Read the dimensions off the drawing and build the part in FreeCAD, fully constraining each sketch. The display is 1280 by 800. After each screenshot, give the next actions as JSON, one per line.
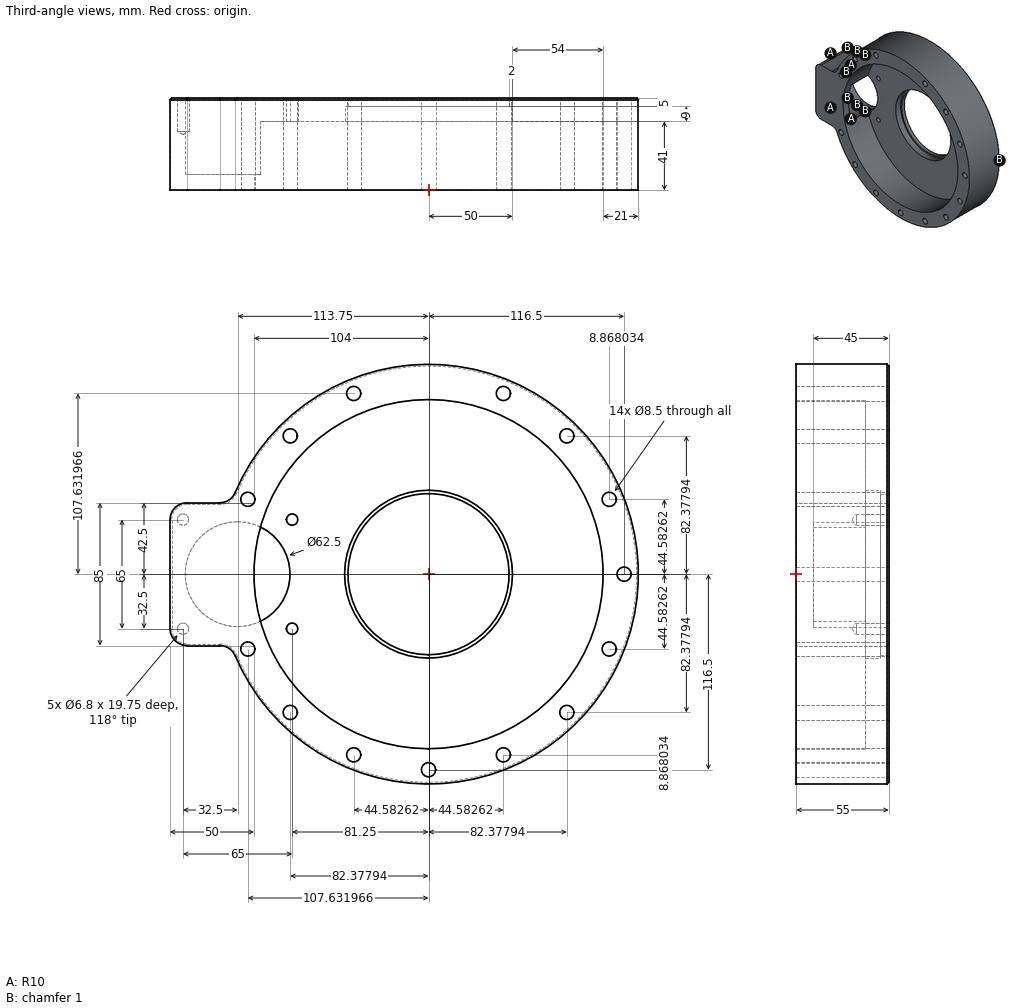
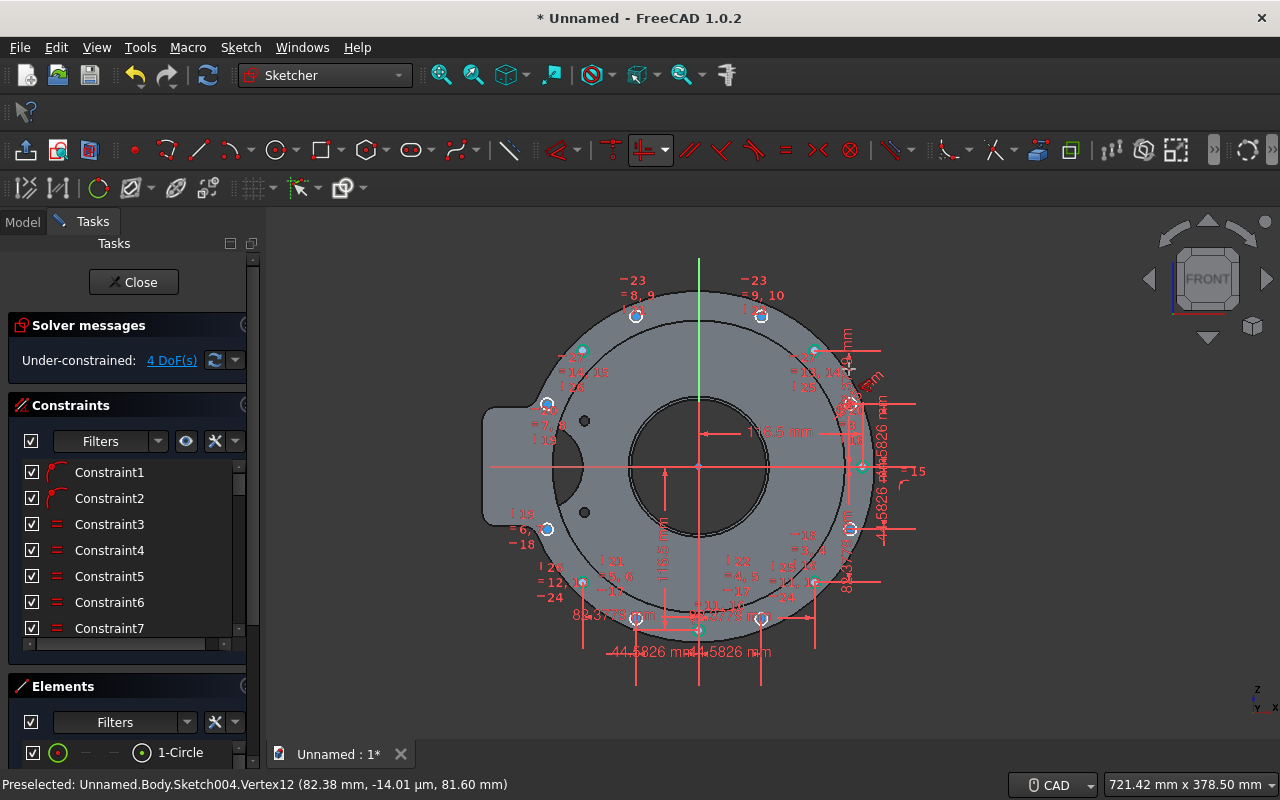
{"action": "scroll", "coordinate": [761, 619], "scroll_direction": "up", "scroll_amount": 6}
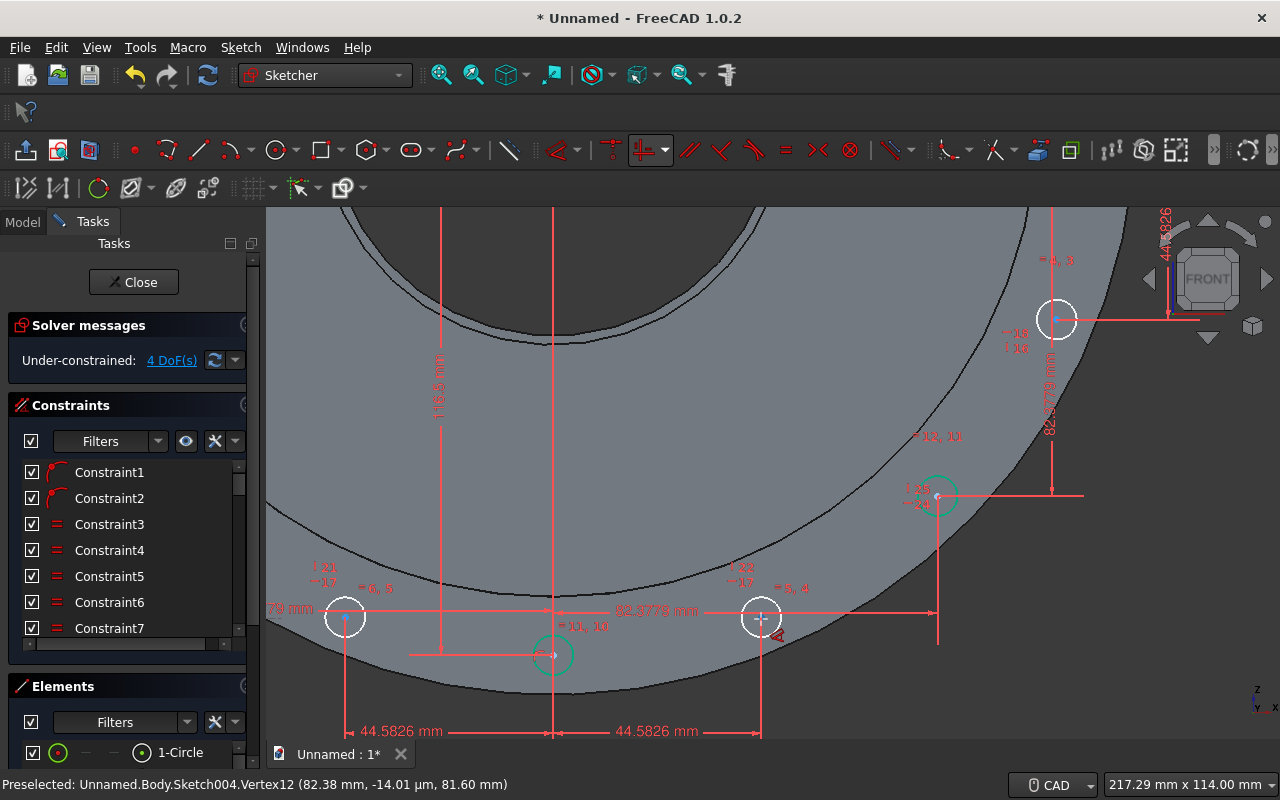
{"action": "left_click", "coordinate": [761, 617]}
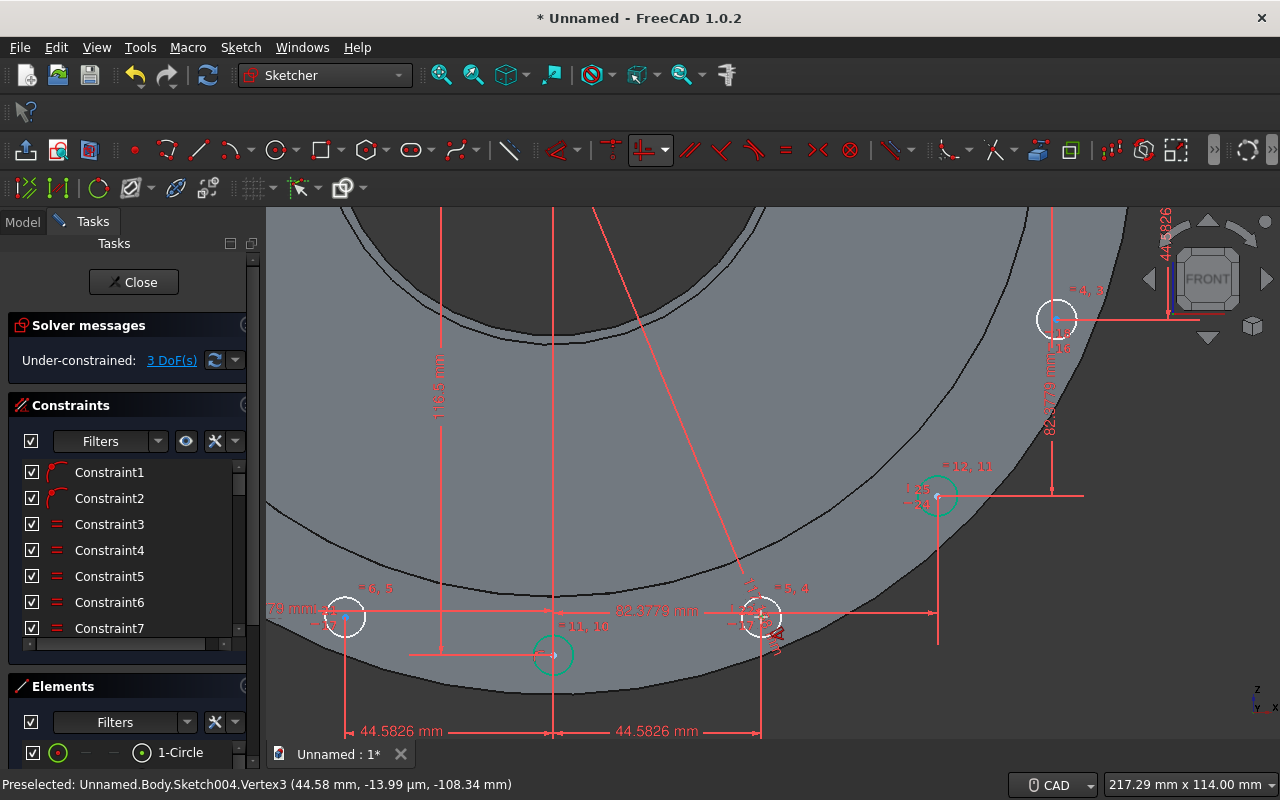
{"action": "left_click", "coordinate": [553, 655]}
{"action": "left_click", "coordinate": [795, 636]}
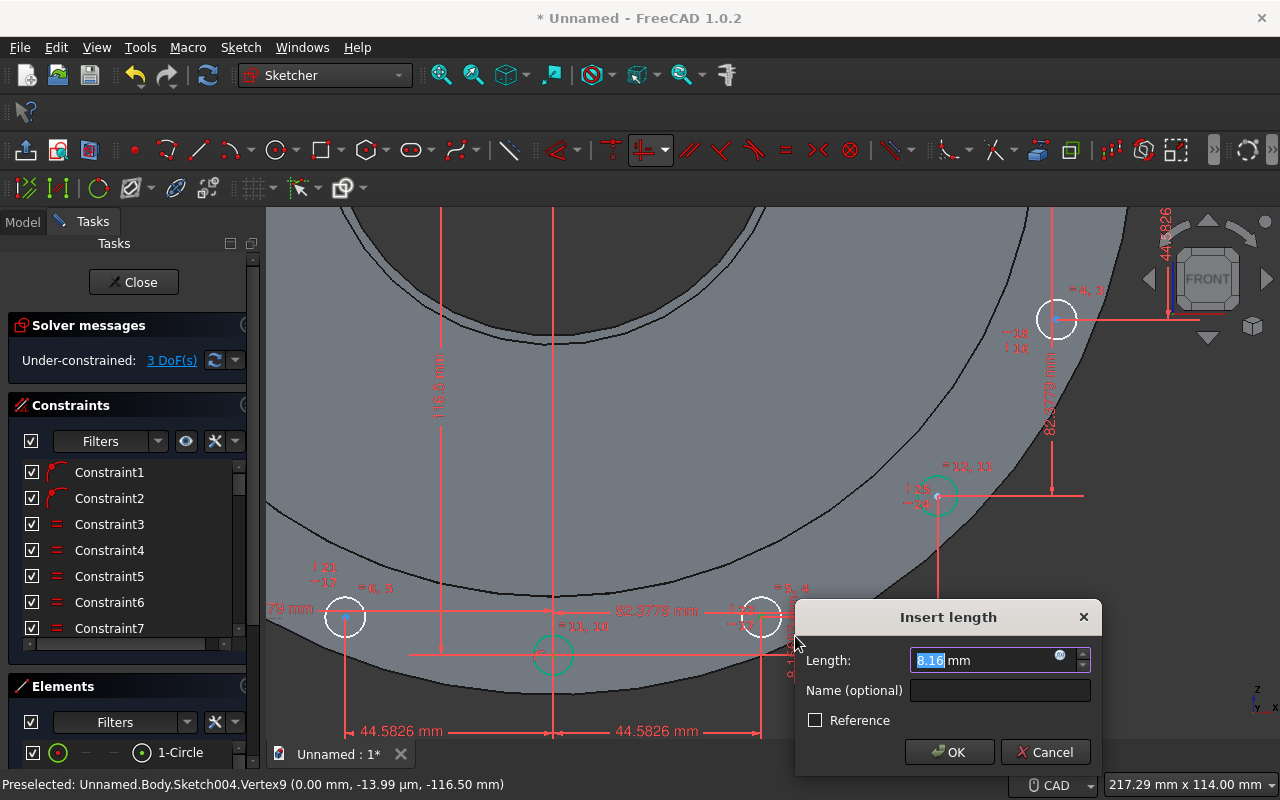
{"action": "type", "text": "8.868034"}
{"action": "key", "text": "Return"}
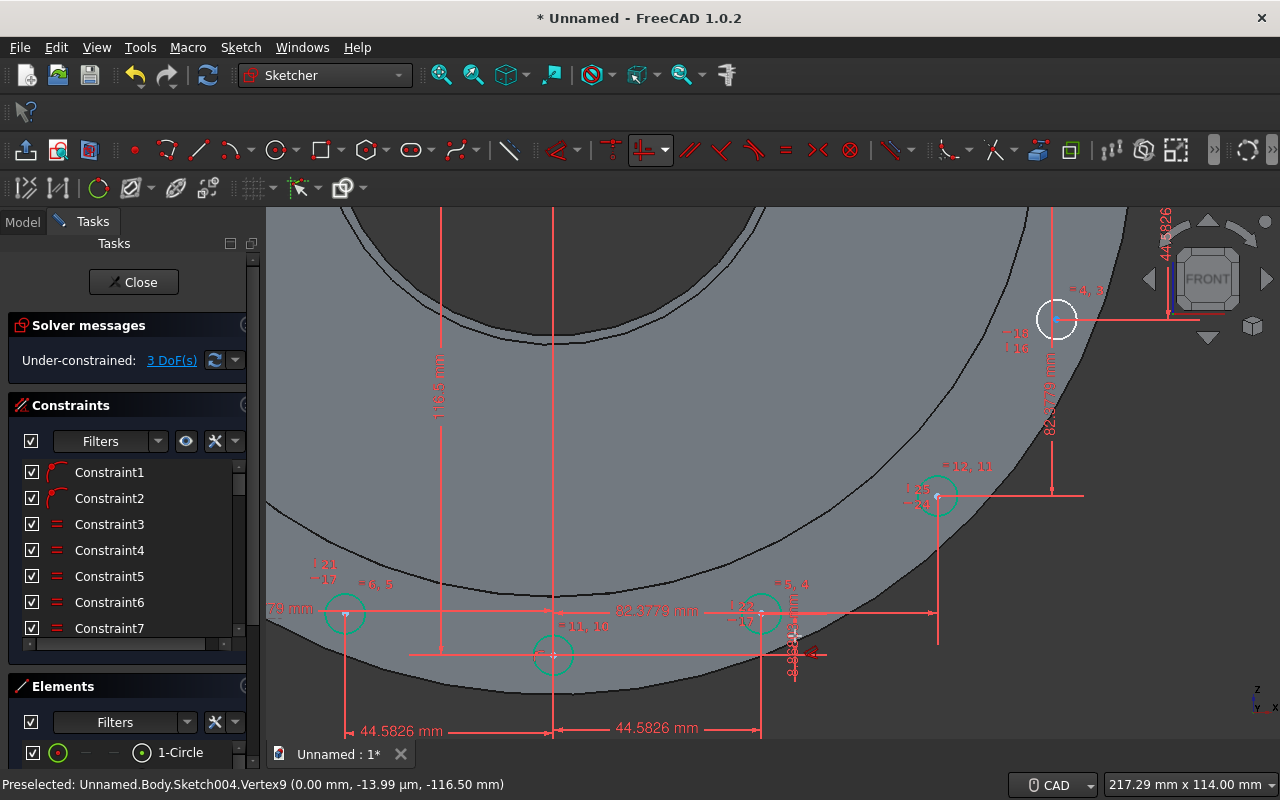
{"action": "scroll", "coordinate": [761, 620], "scroll_direction": "down", "scroll_amount": 6}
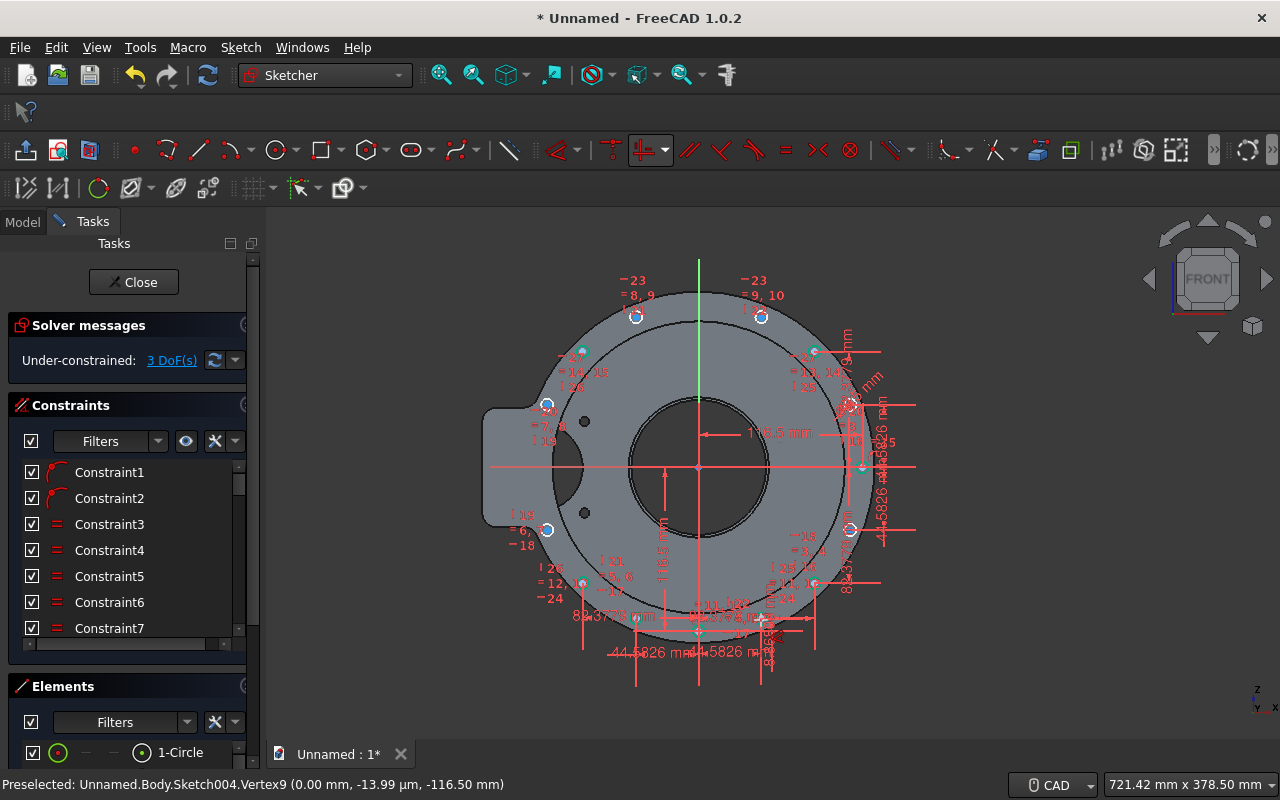
{"action": "scroll", "coordinate": [850, 405], "scroll_direction": "up", "scroll_amount": 6}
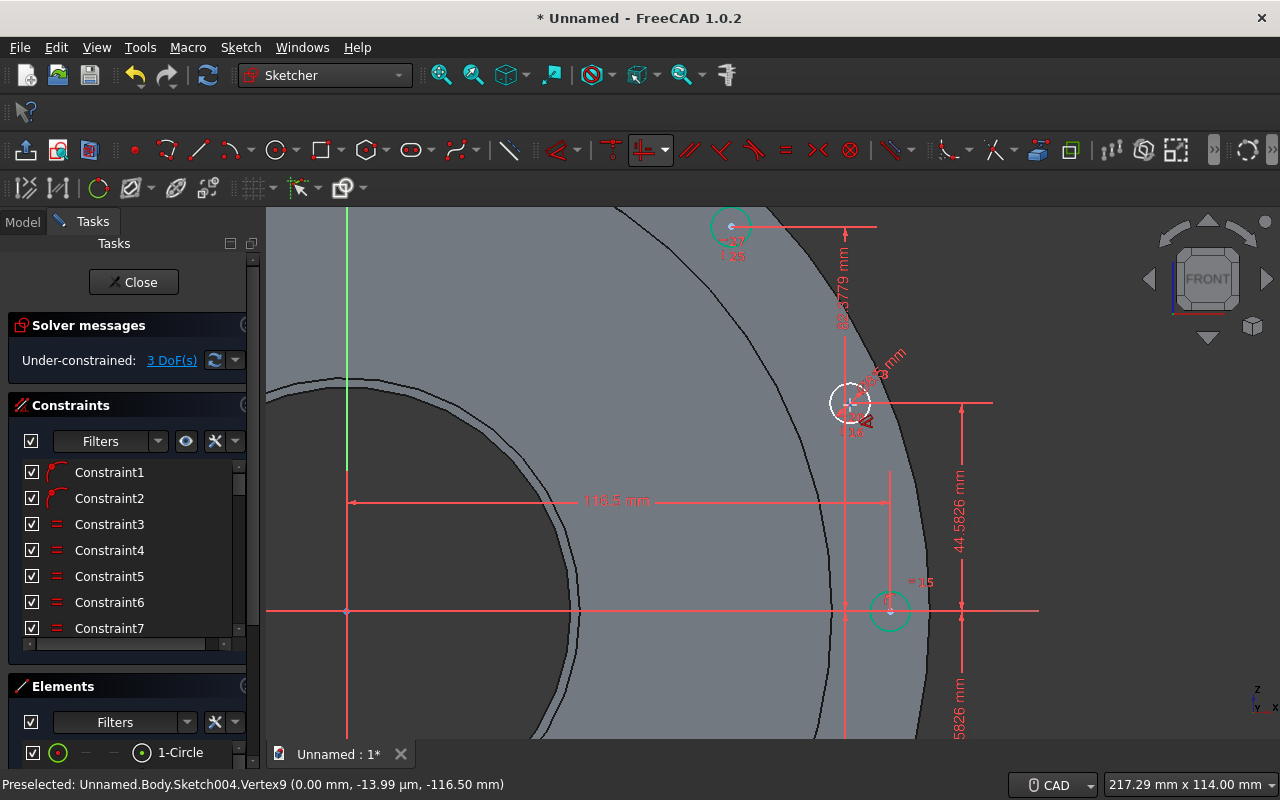
{"action": "left_click", "coordinate": [850, 403]}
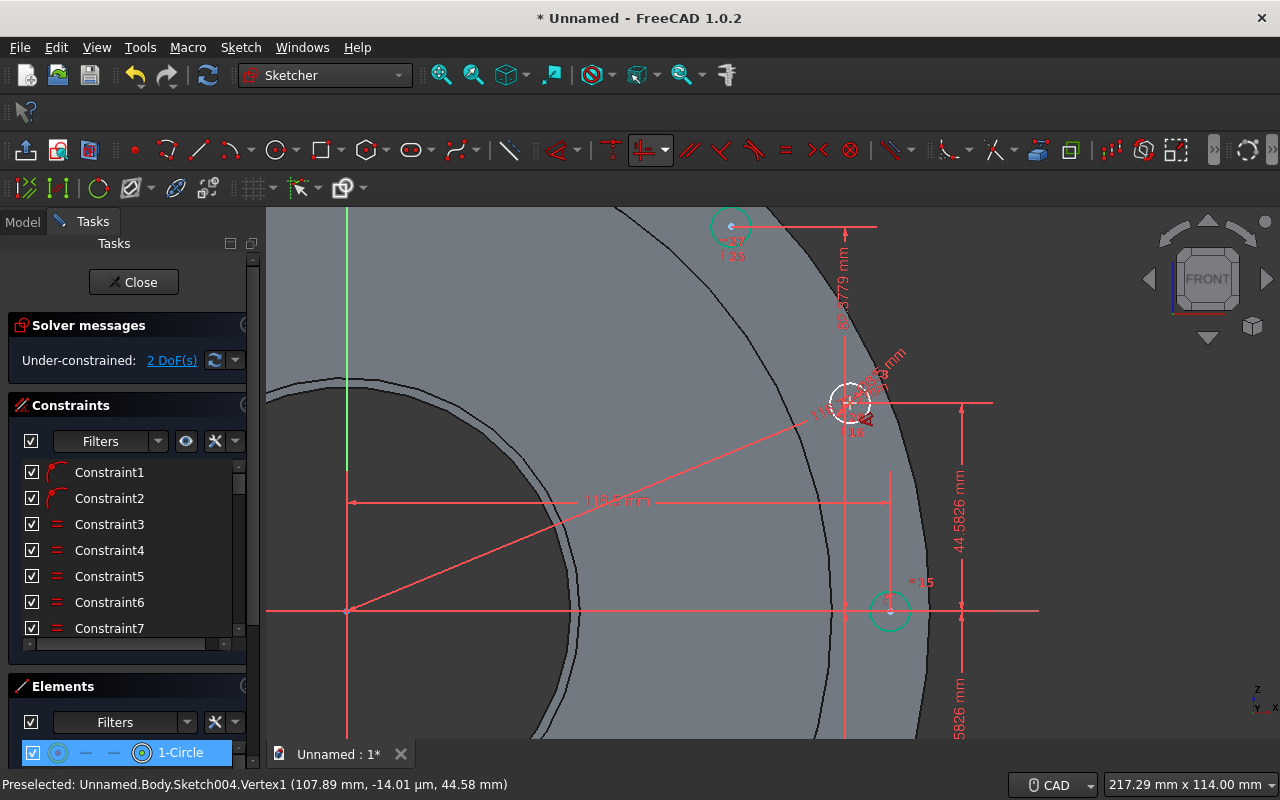
{"action": "left_click", "coordinate": [890, 611]}
{"action": "left_click", "coordinate": [870, 645]}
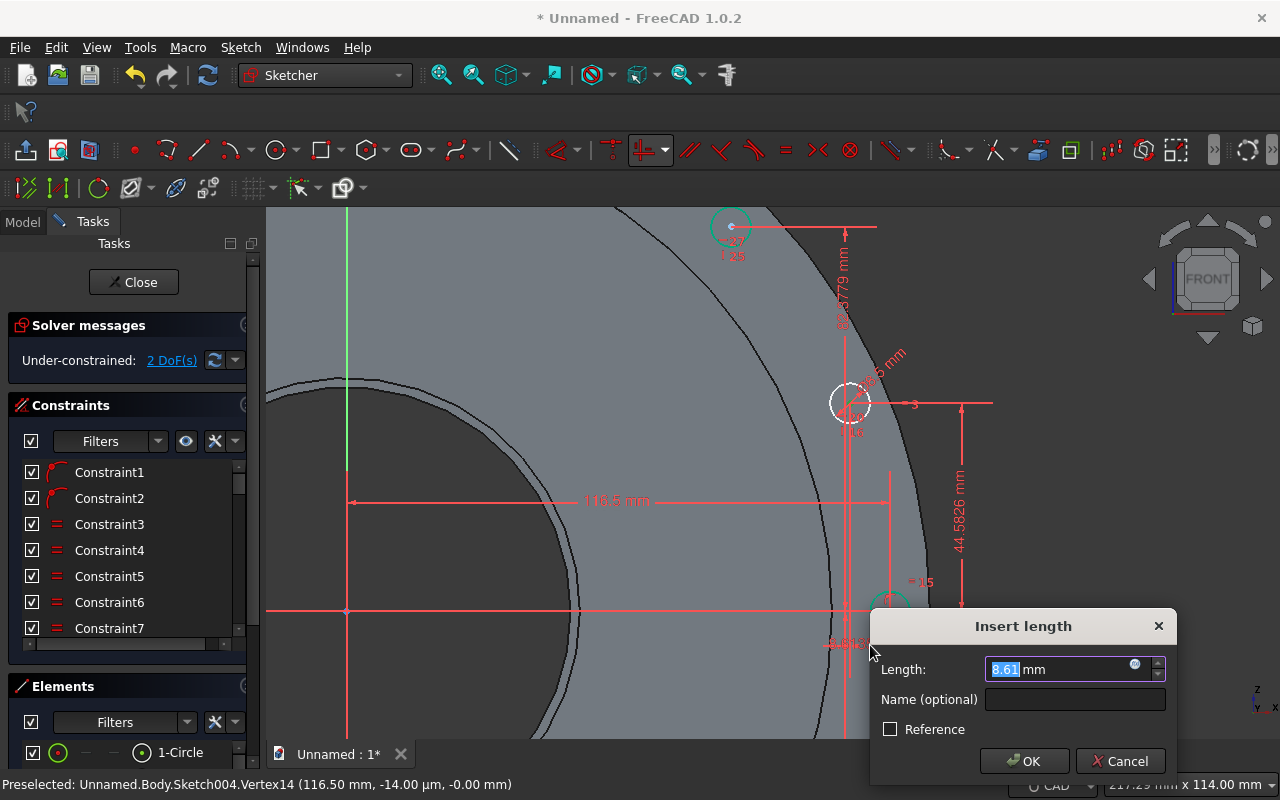
{"action": "type", "text": "8.868034"}
{"action": "key", "text": "Return"}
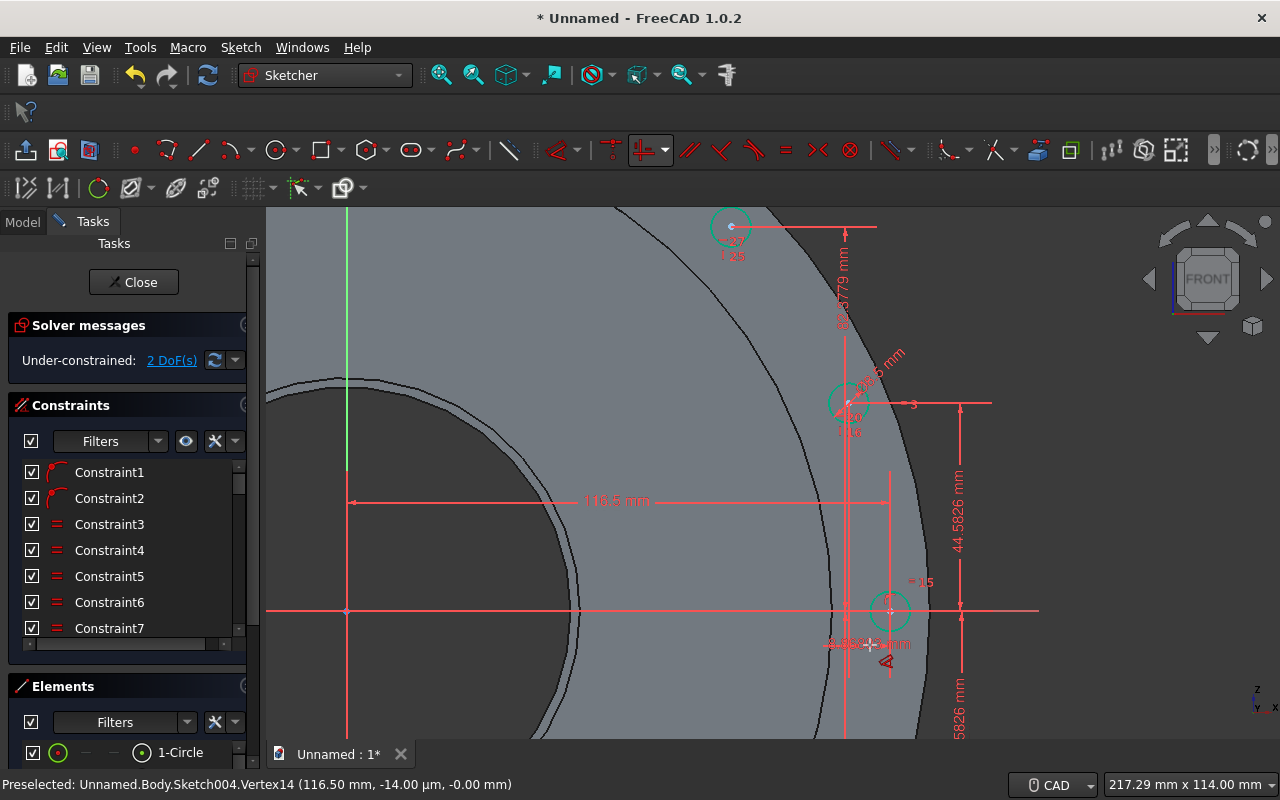
{"action": "scroll", "coordinate": [850, 404], "scroll_direction": "down", "scroll_amount": 6}